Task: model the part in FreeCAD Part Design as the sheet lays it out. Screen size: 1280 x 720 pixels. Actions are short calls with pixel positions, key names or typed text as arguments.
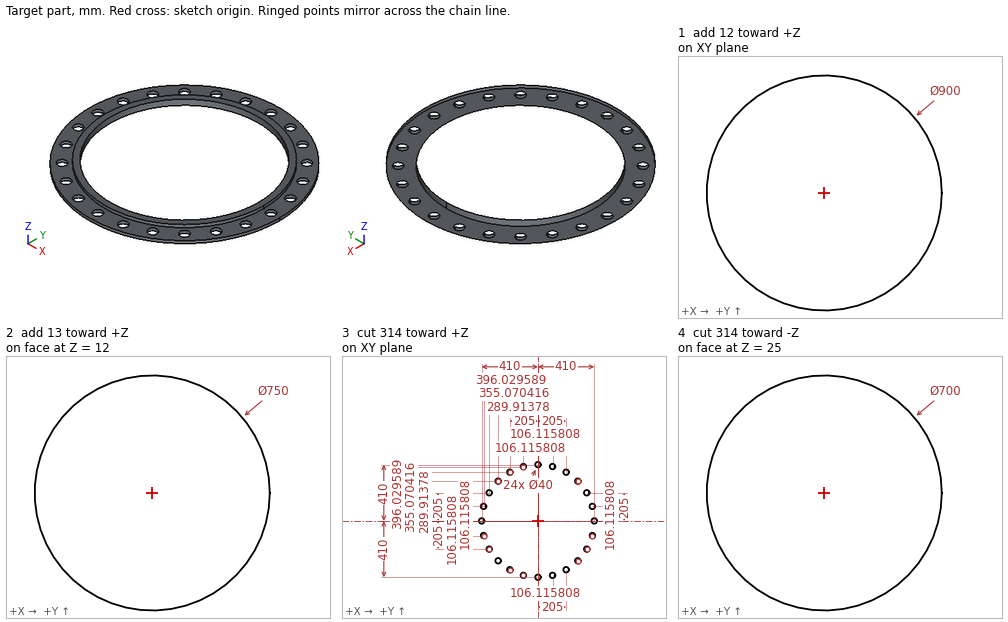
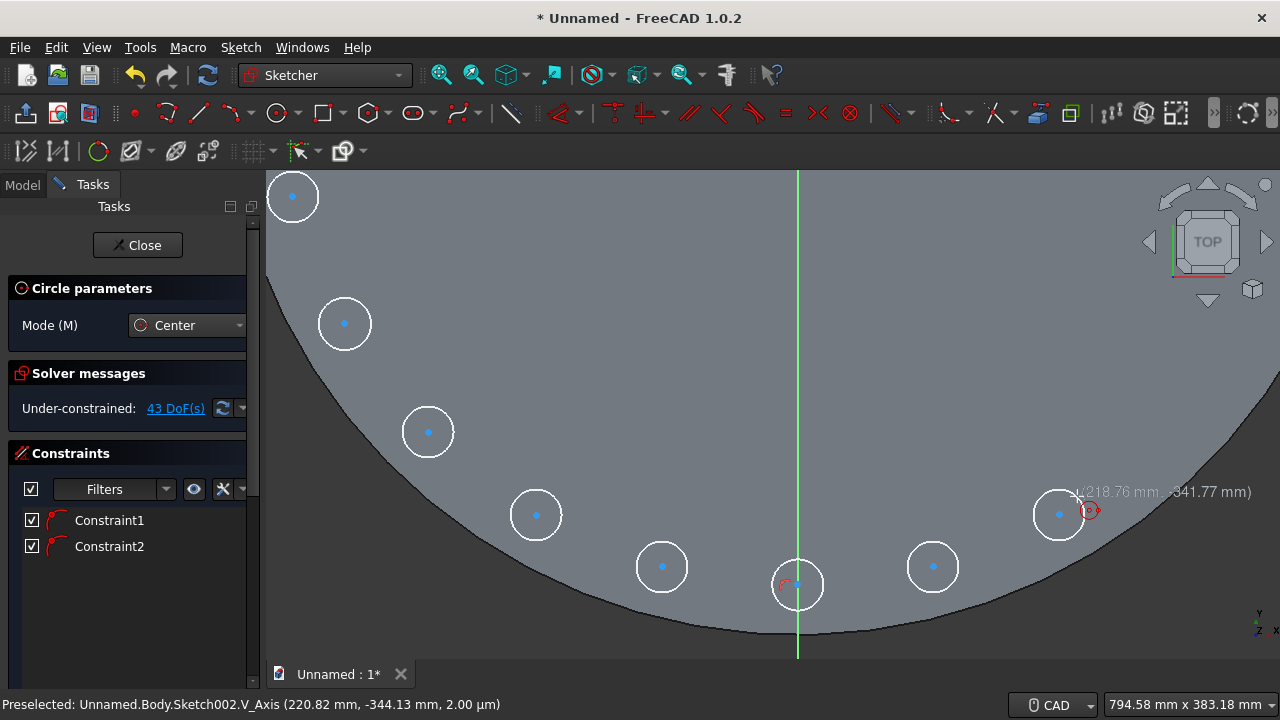
scroll(664, 567, down, 6)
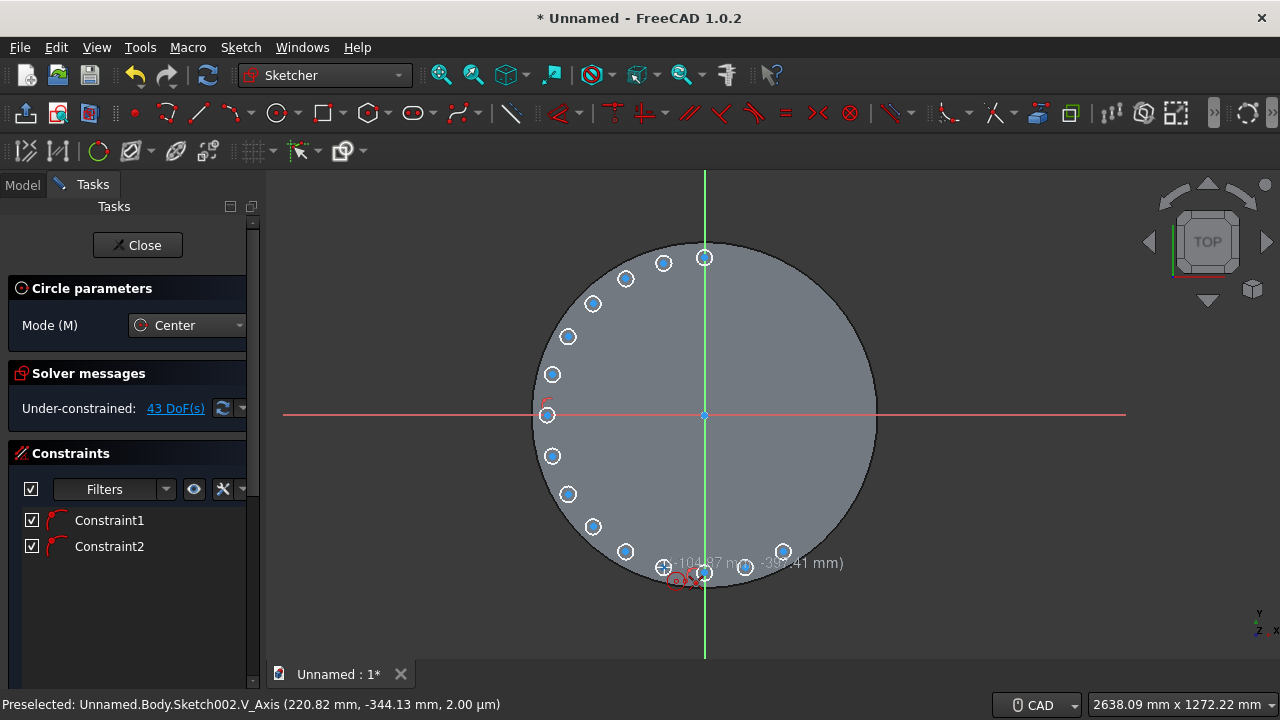
scroll(816, 527, up, 6)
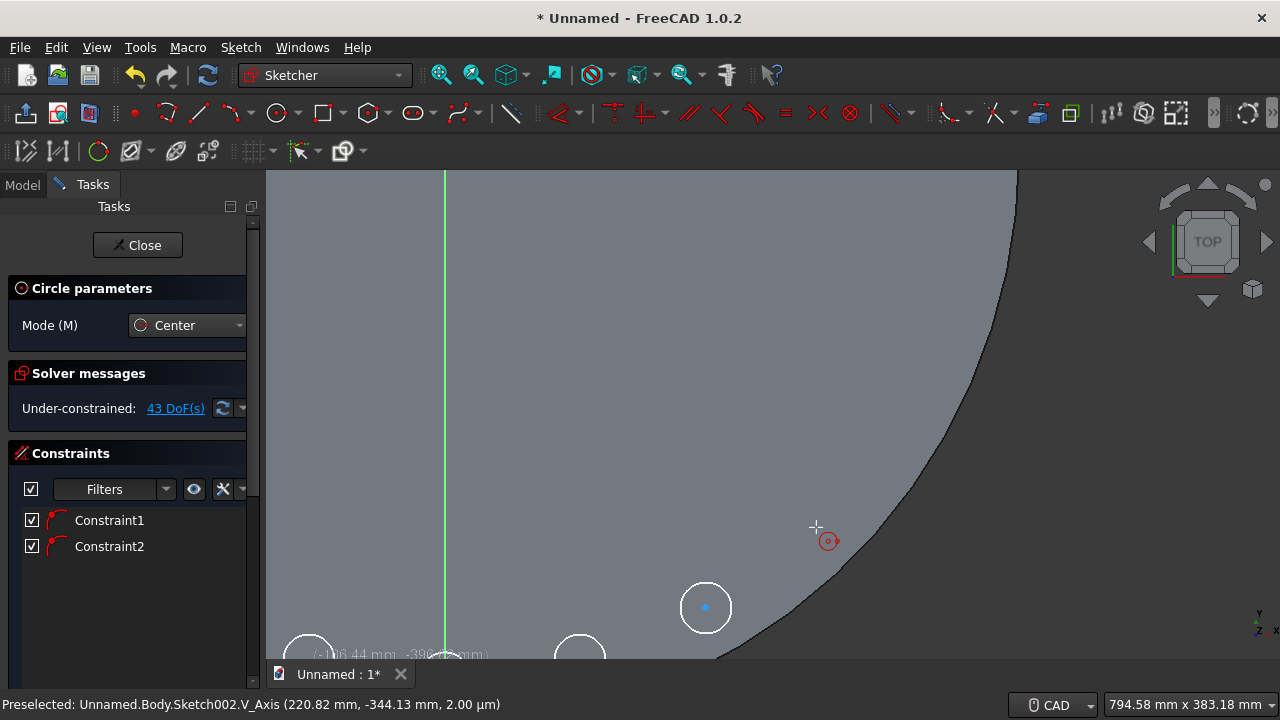
click(815, 524)
click(833, 506)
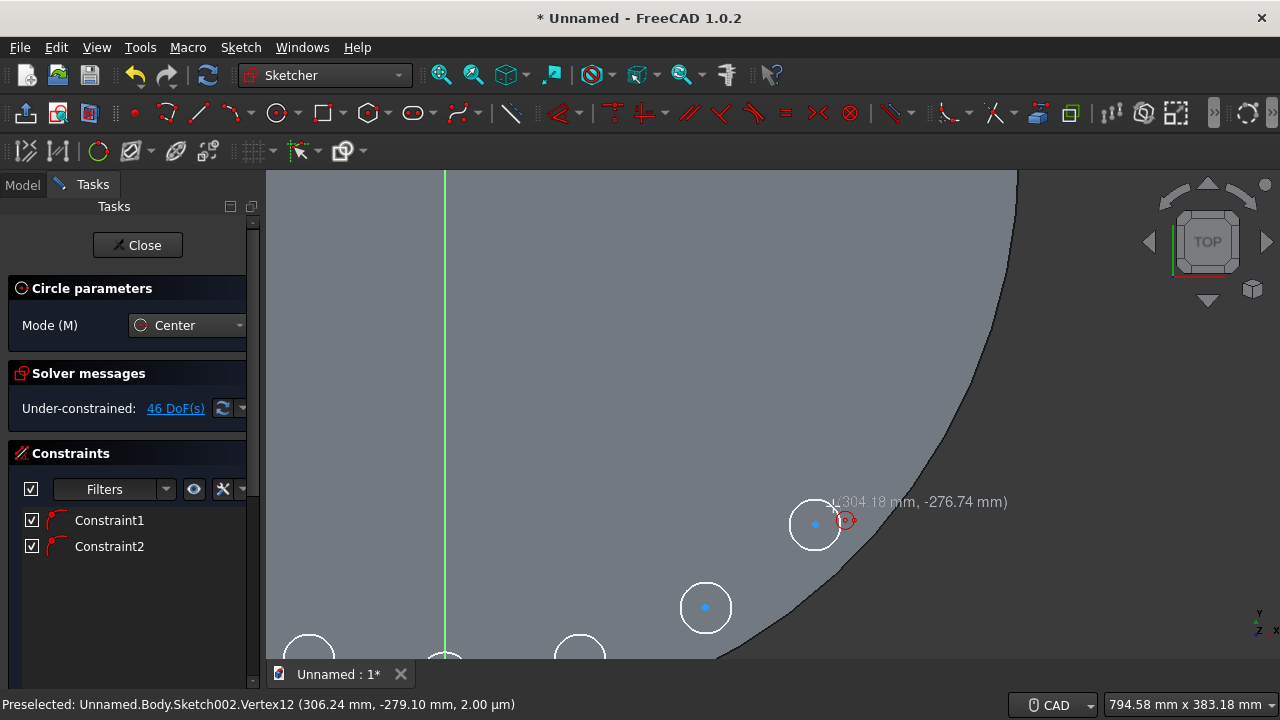
click(898, 415)
click(916, 397)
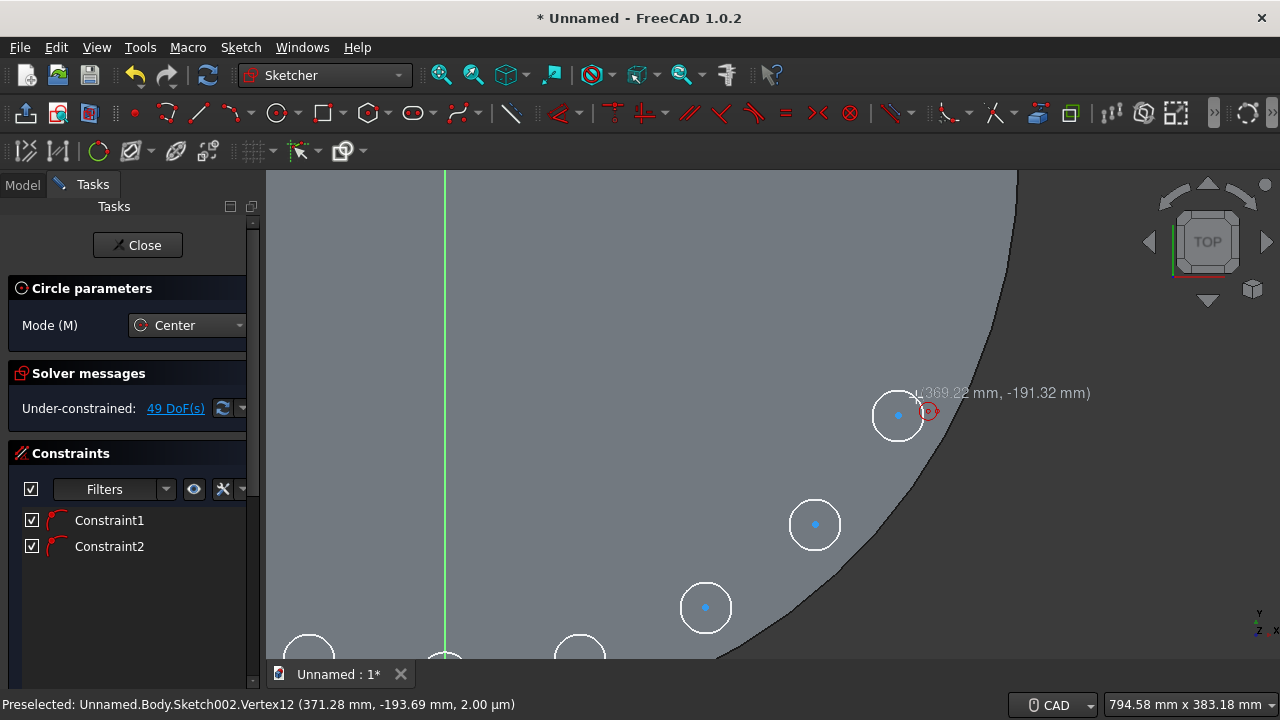
click(950, 289)
click(968, 271)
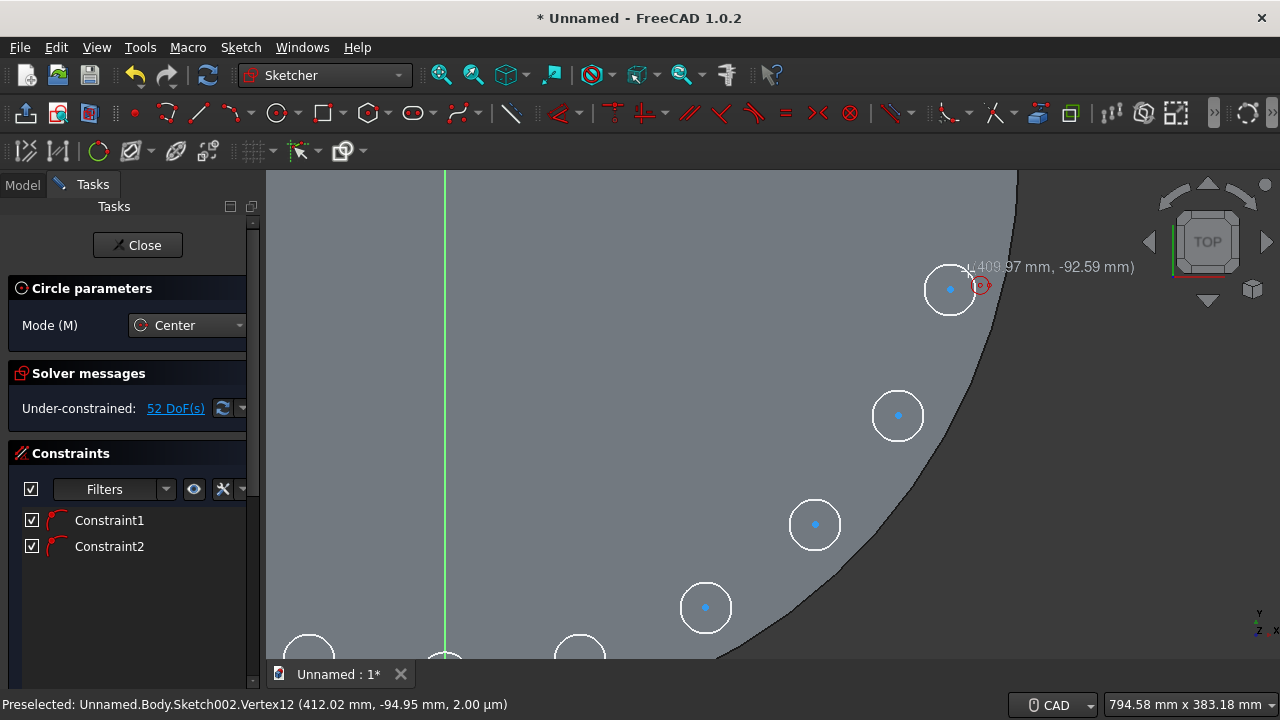
scroll(816, 527, down, 6)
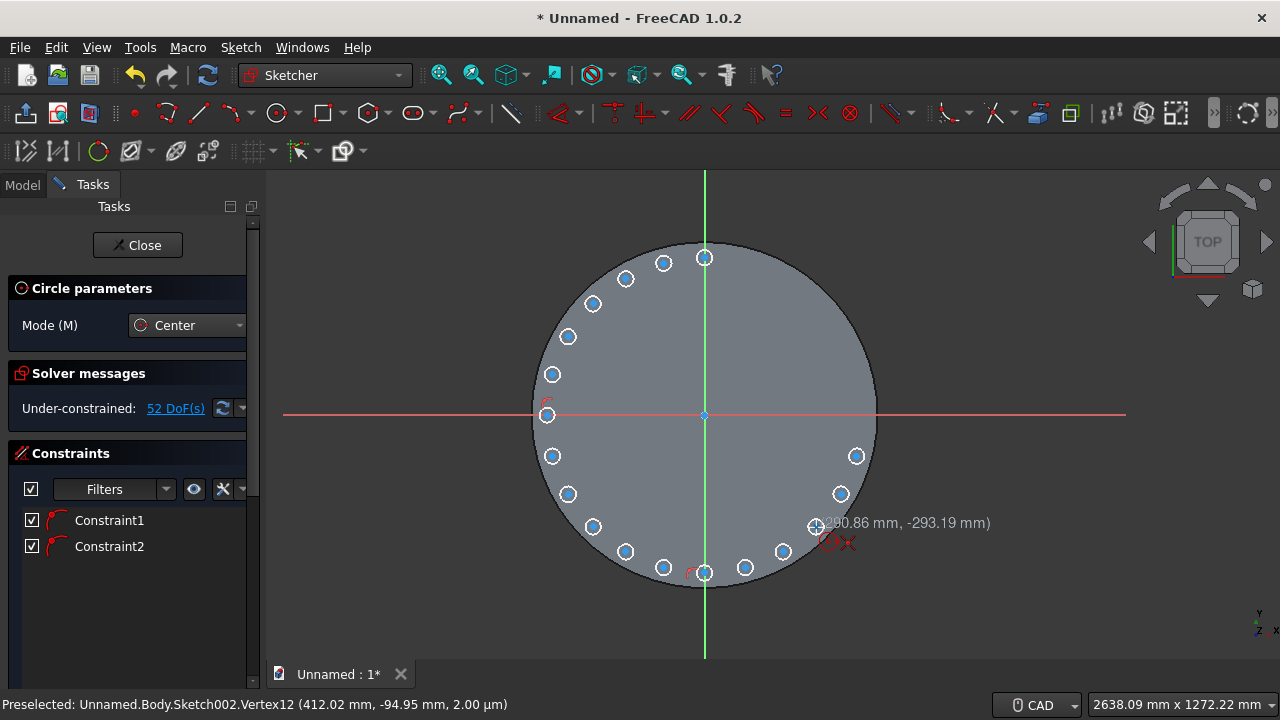
scroll(862, 415, up, 6)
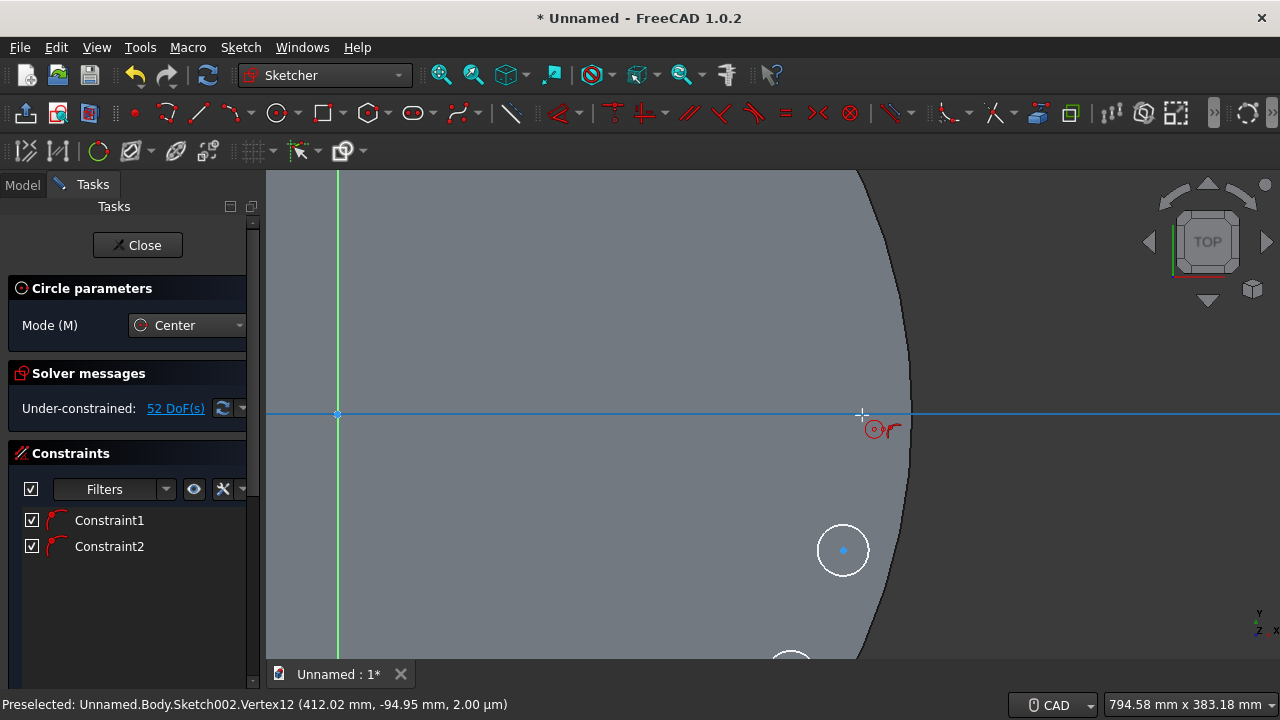
click(861, 414)
click(879, 396)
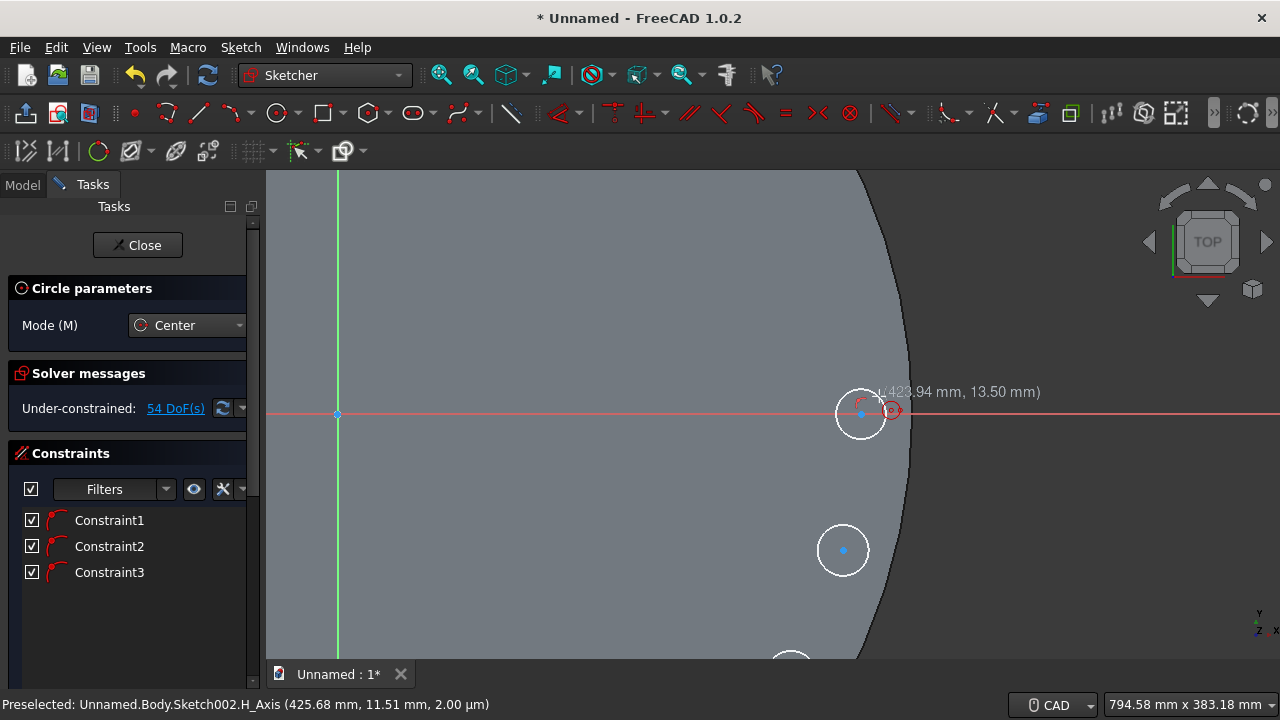
click(843, 279)
click(861, 261)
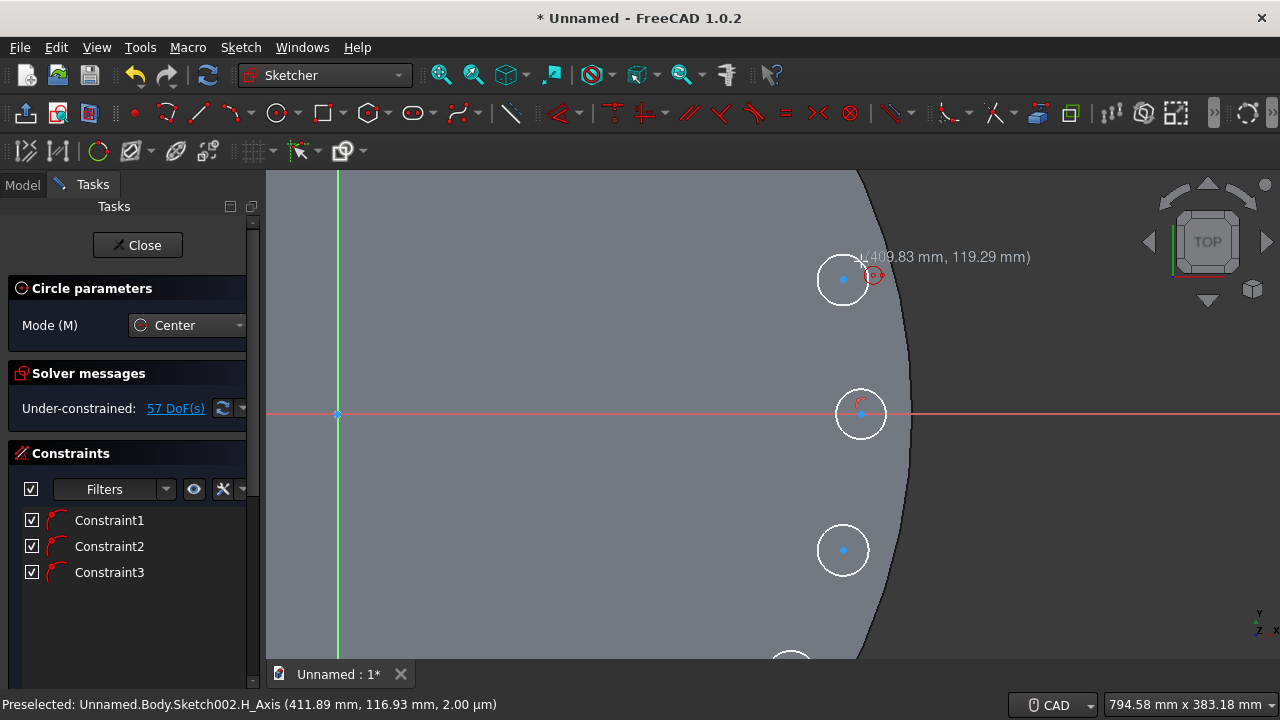
scroll(862, 415, down, 6)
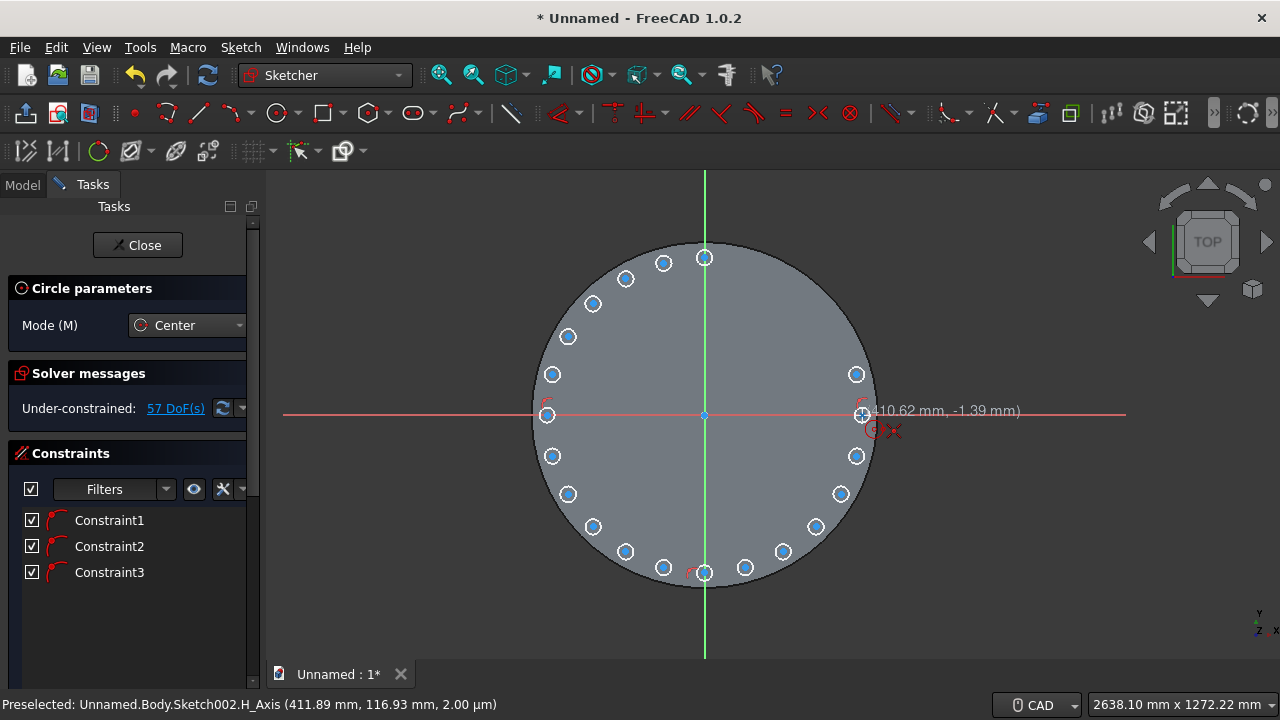
scroll(841, 336, up, 6)